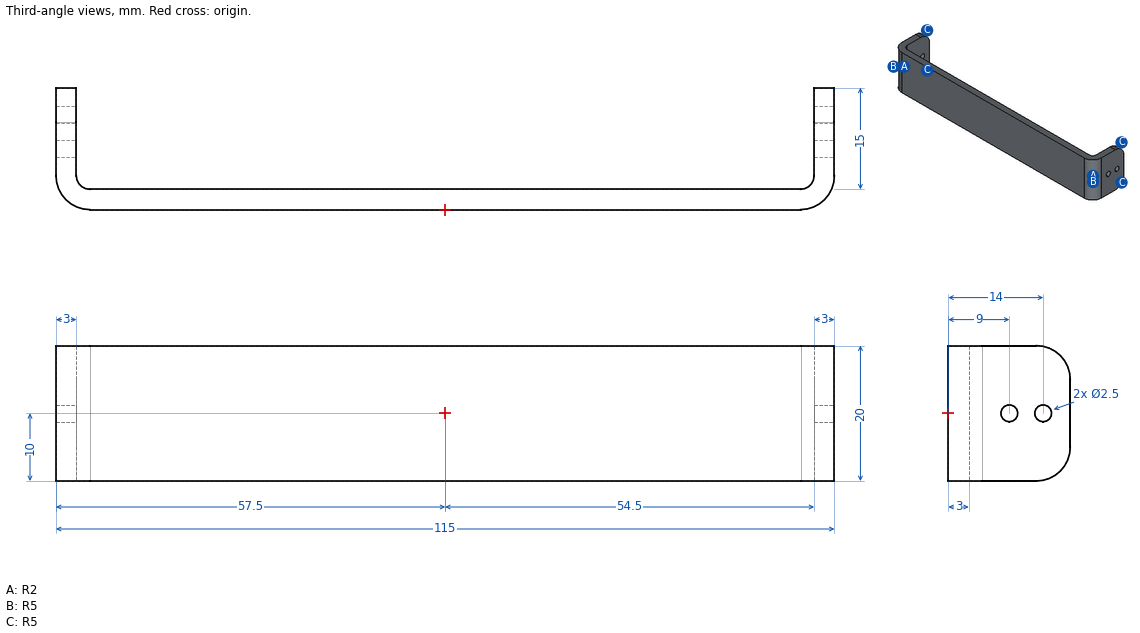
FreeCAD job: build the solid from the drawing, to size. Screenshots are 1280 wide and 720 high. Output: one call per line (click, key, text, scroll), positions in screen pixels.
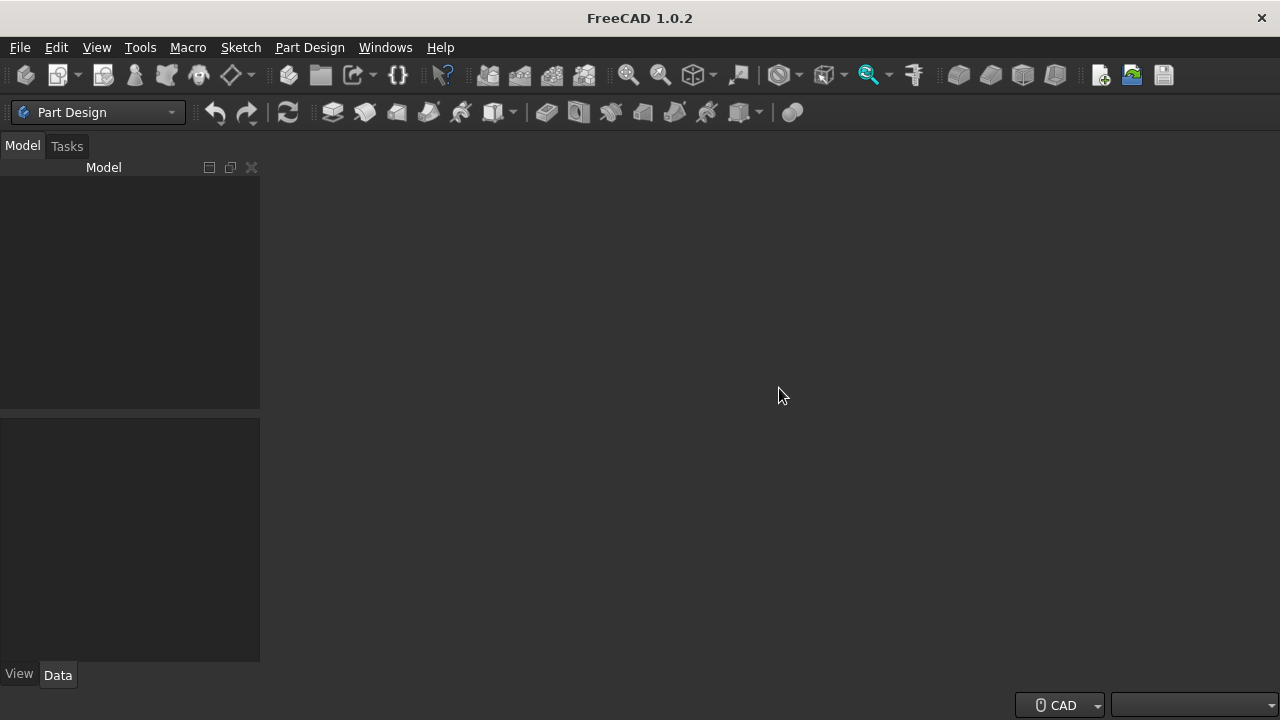
click(1100, 76)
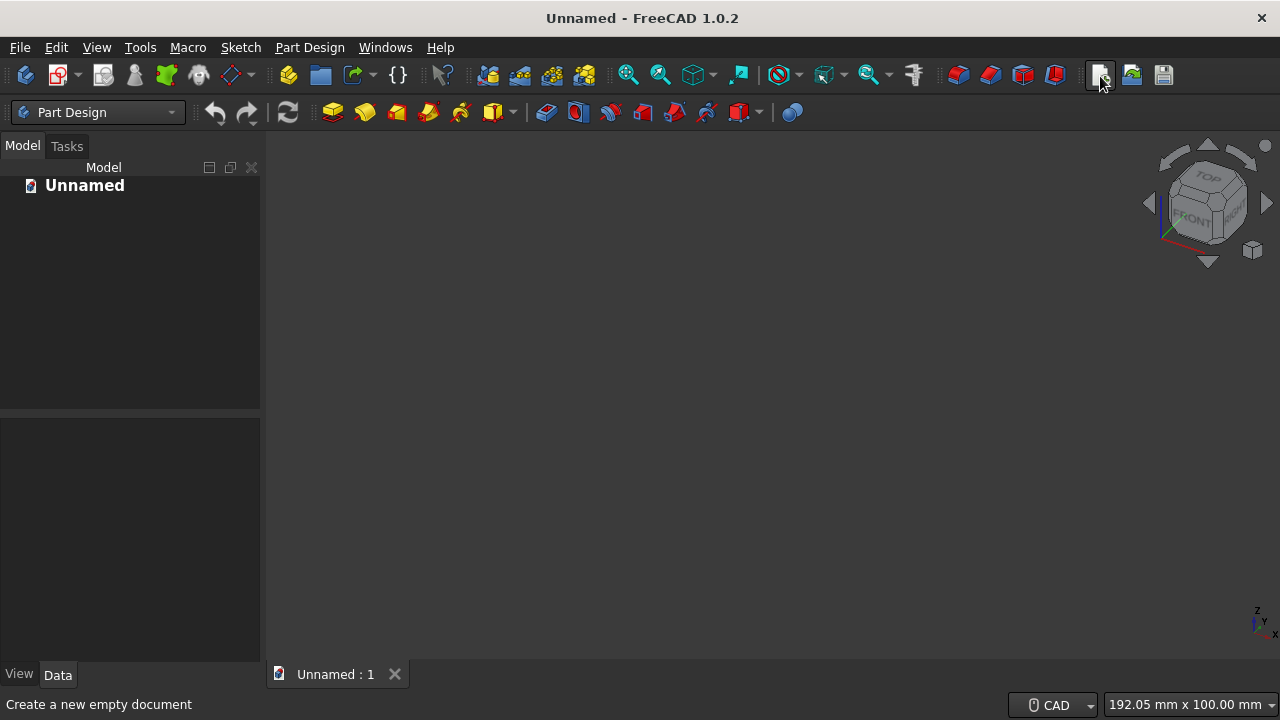
click(58, 76)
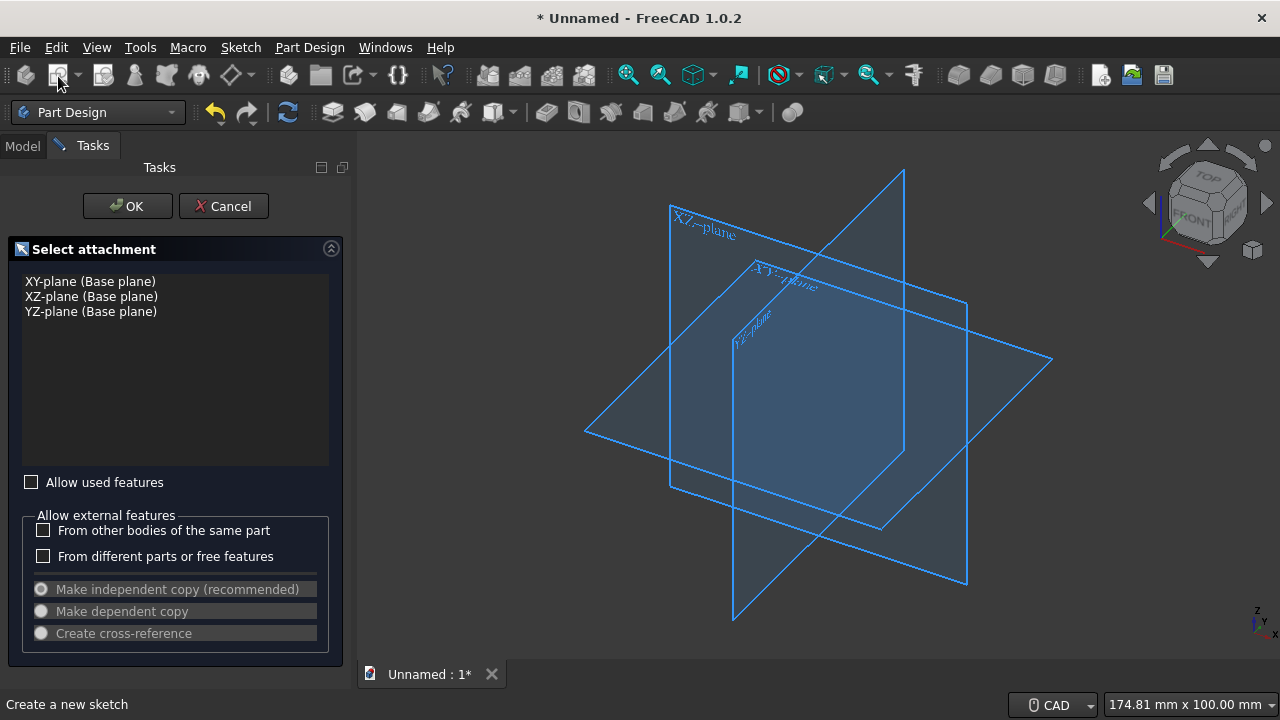
click(82, 296)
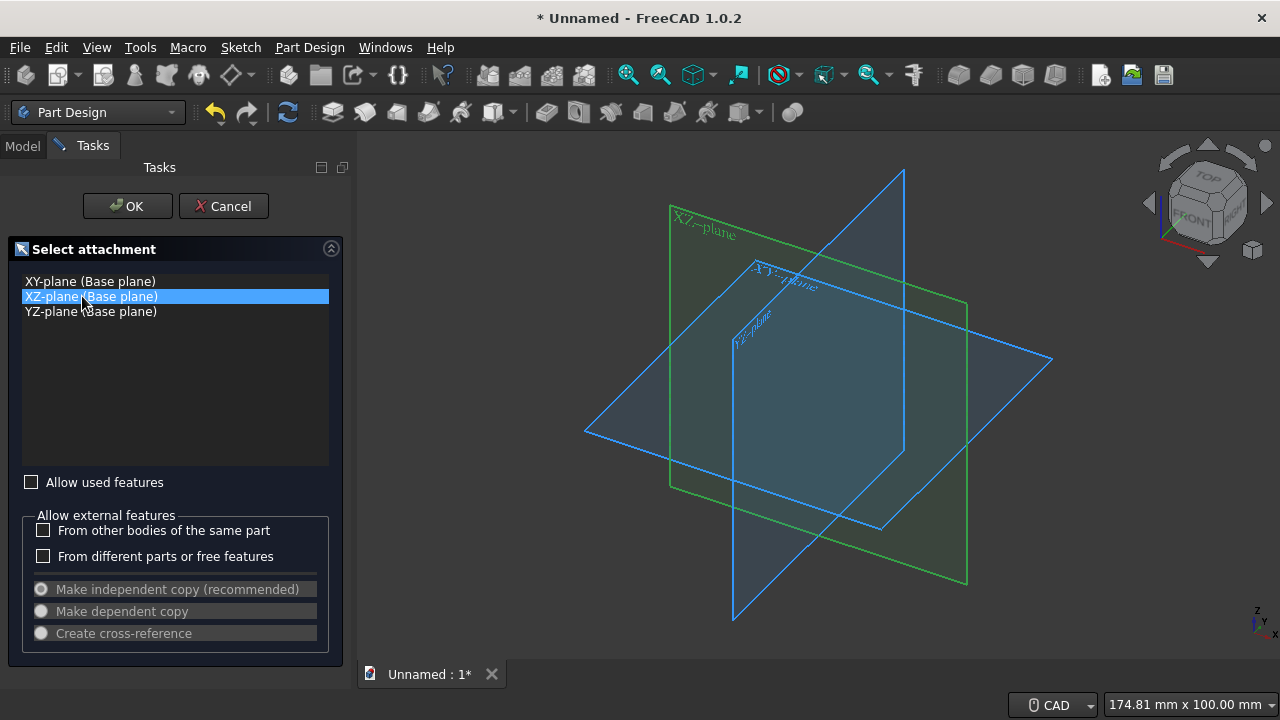
click(128, 206)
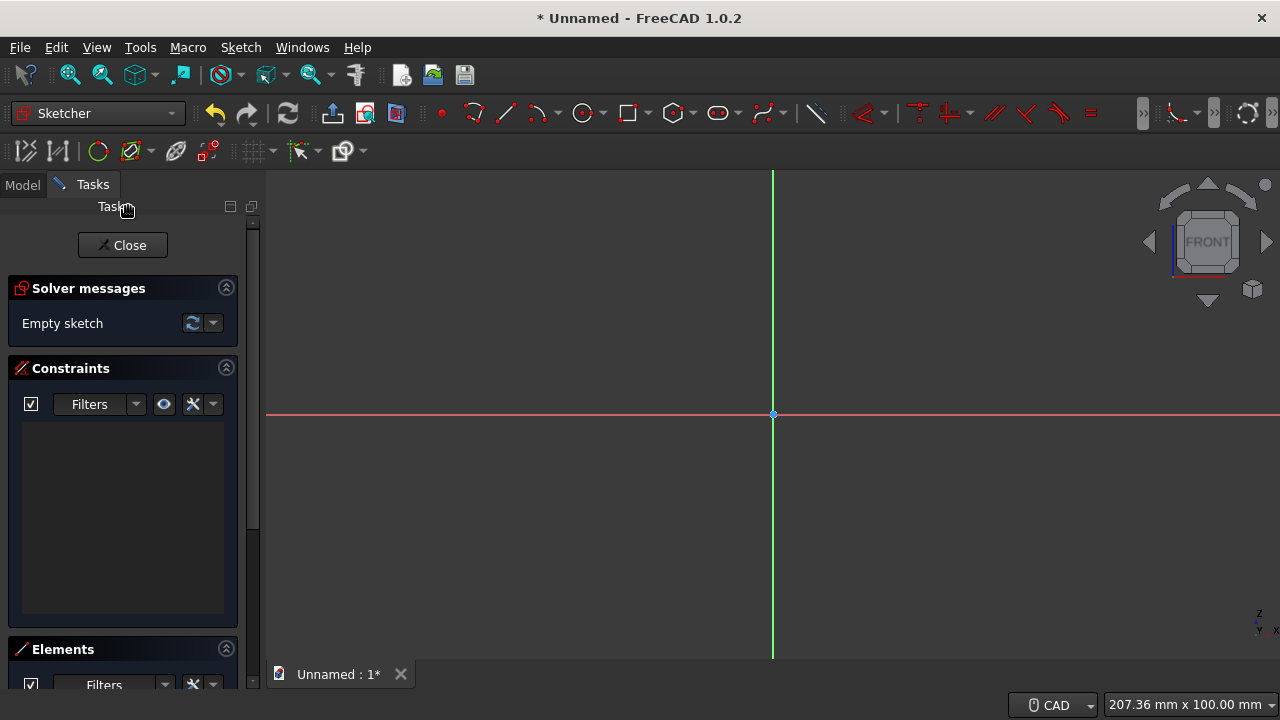
key(g)
key(v)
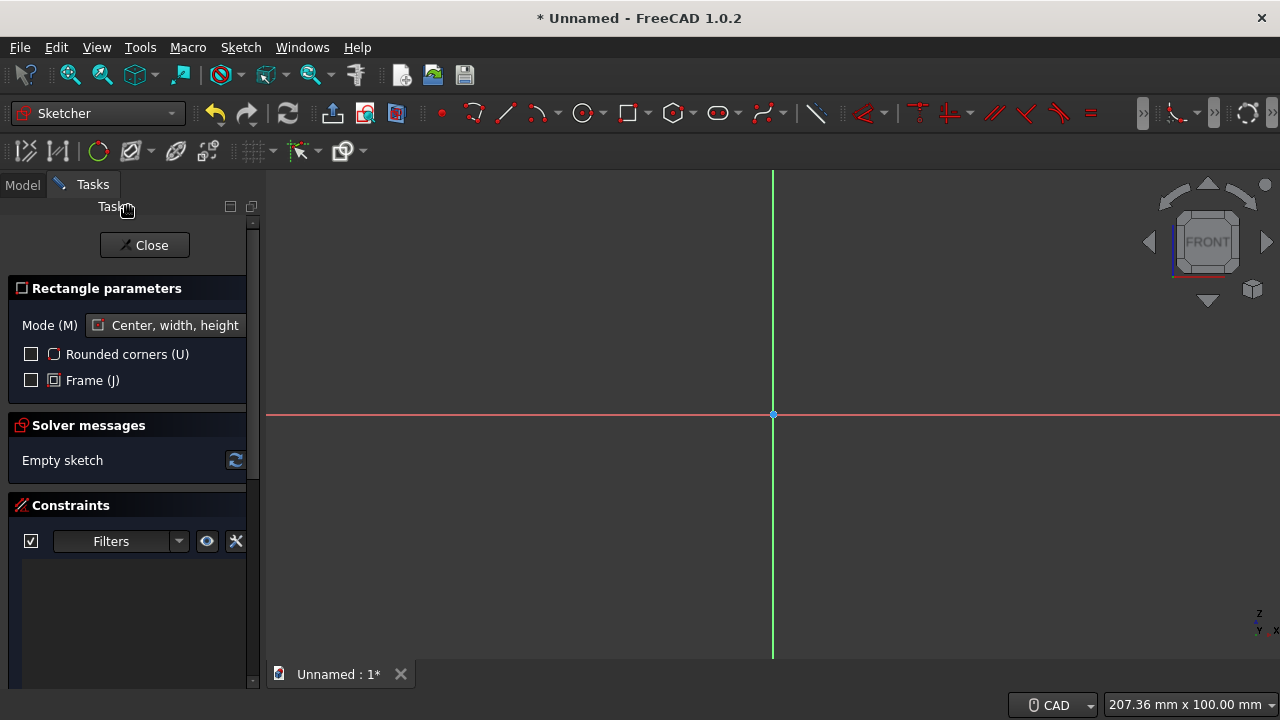
click(773, 414)
move(1054, 366)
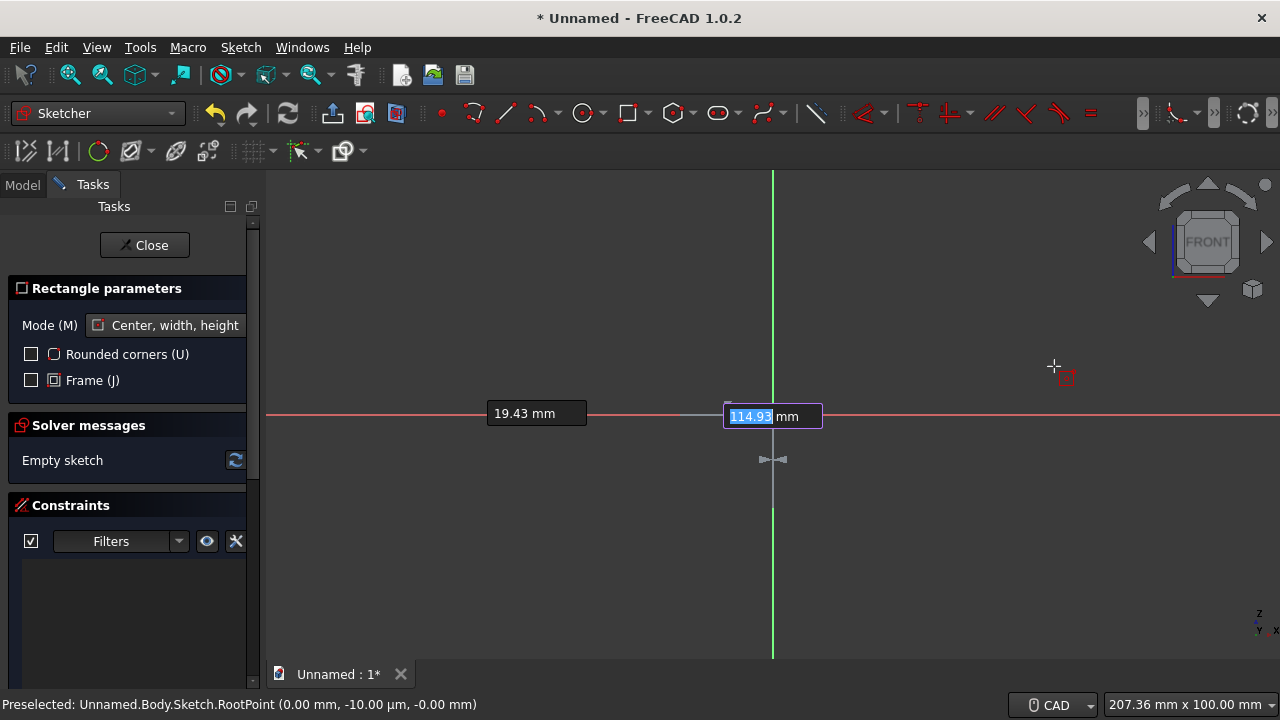
text(115)
key(Tab)
text(20)
key(Return)
key(Escape)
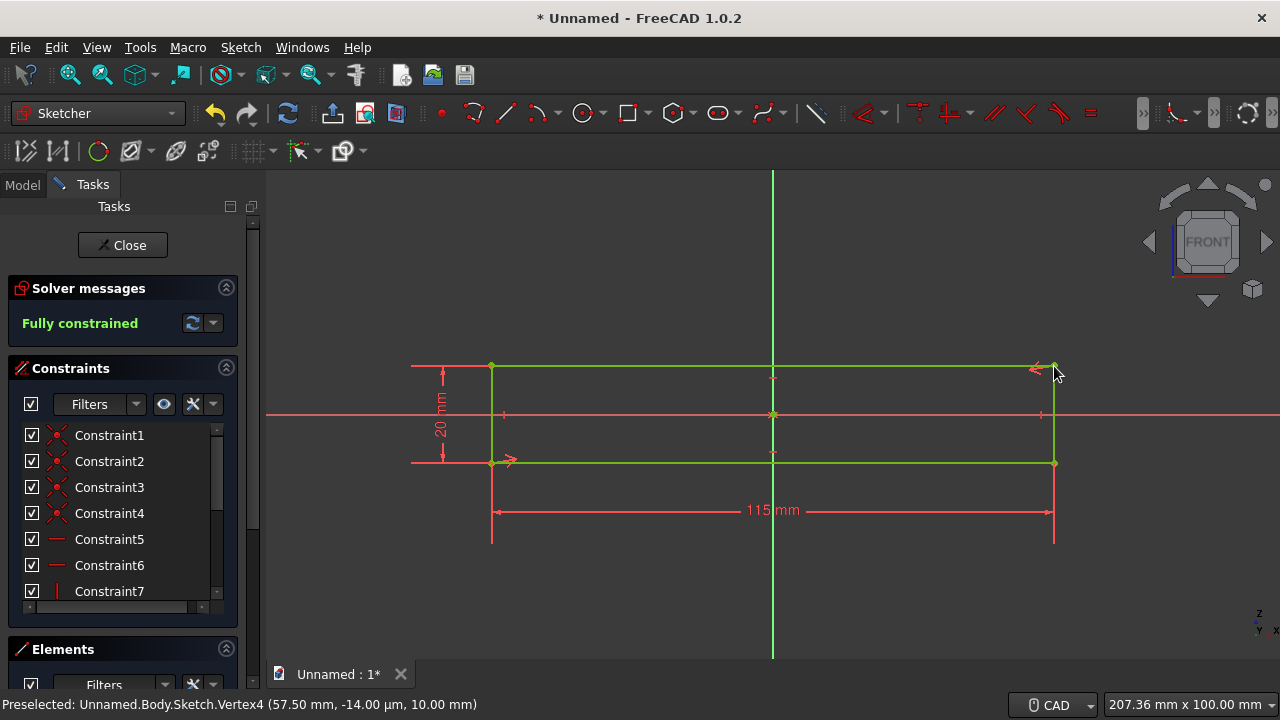
click(123, 245)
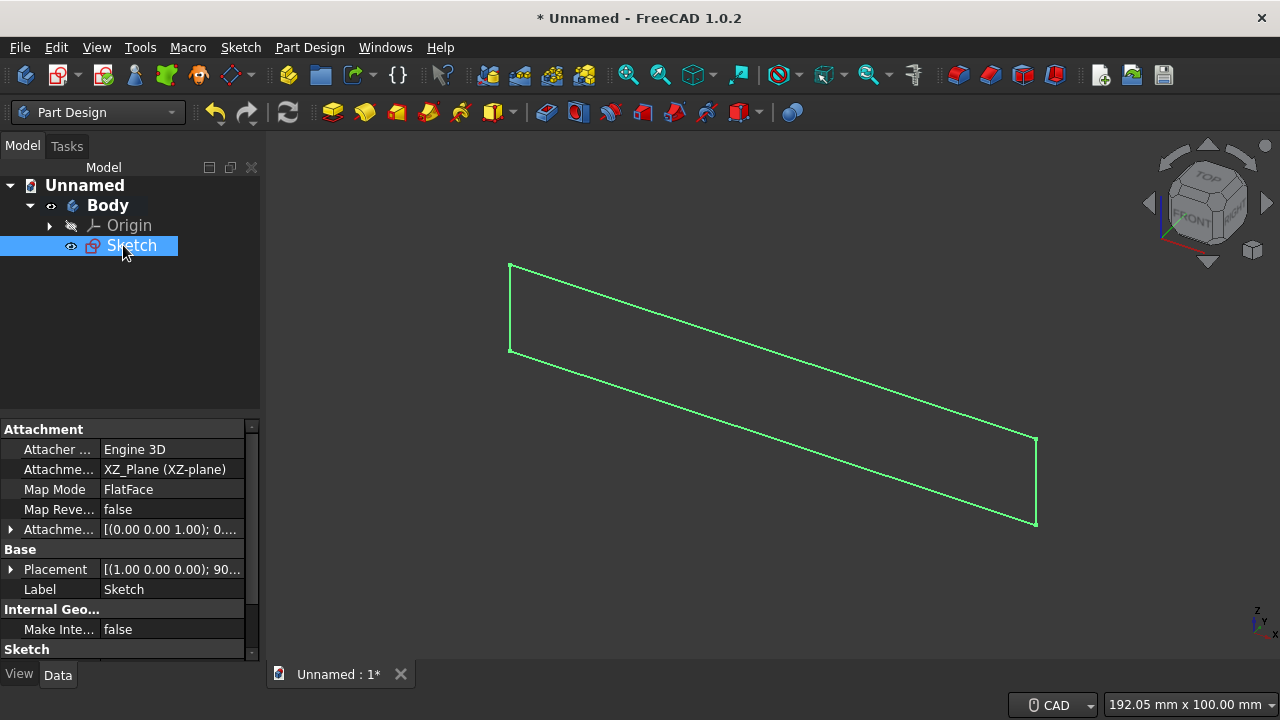
click(334, 112)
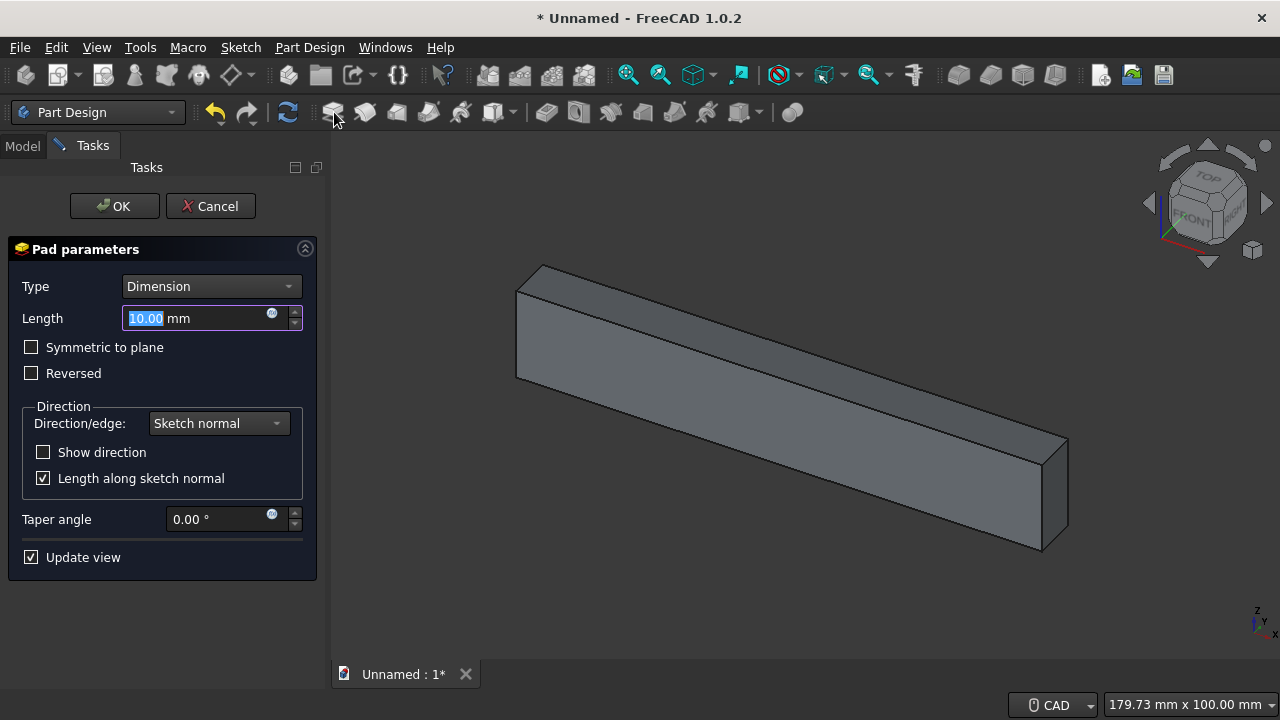
text(3)
key(Tab)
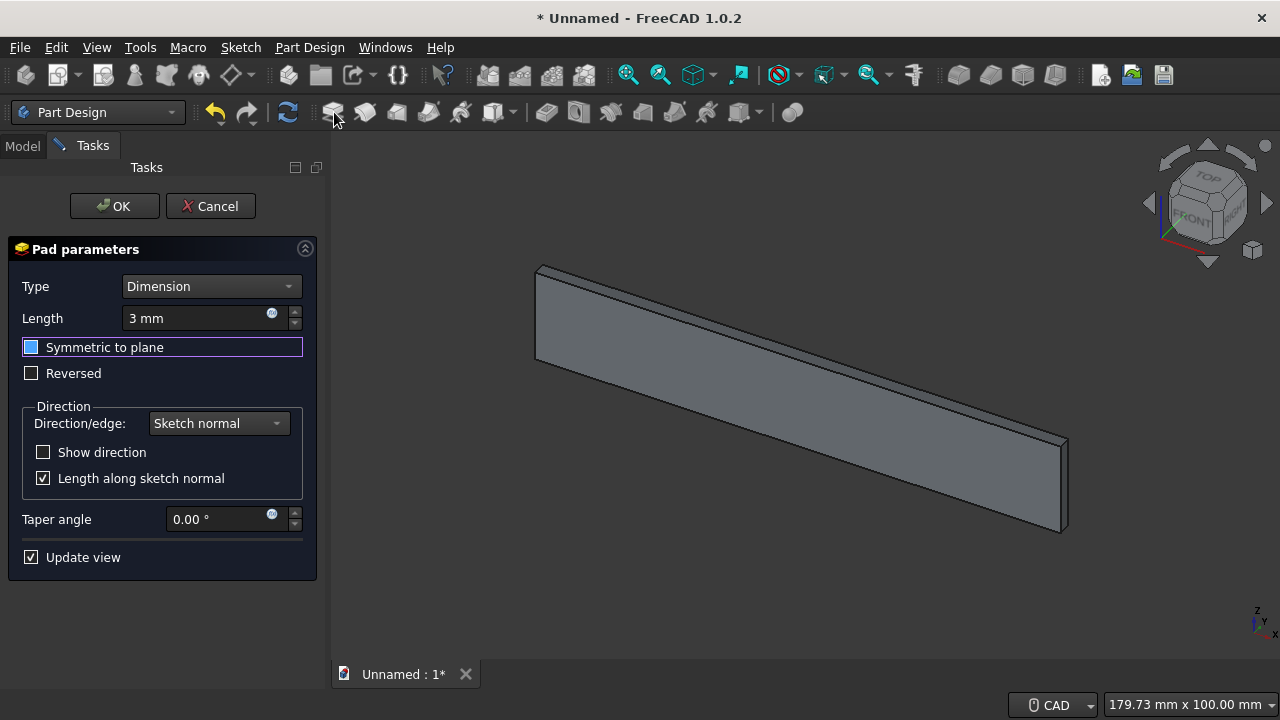
click(30, 373)